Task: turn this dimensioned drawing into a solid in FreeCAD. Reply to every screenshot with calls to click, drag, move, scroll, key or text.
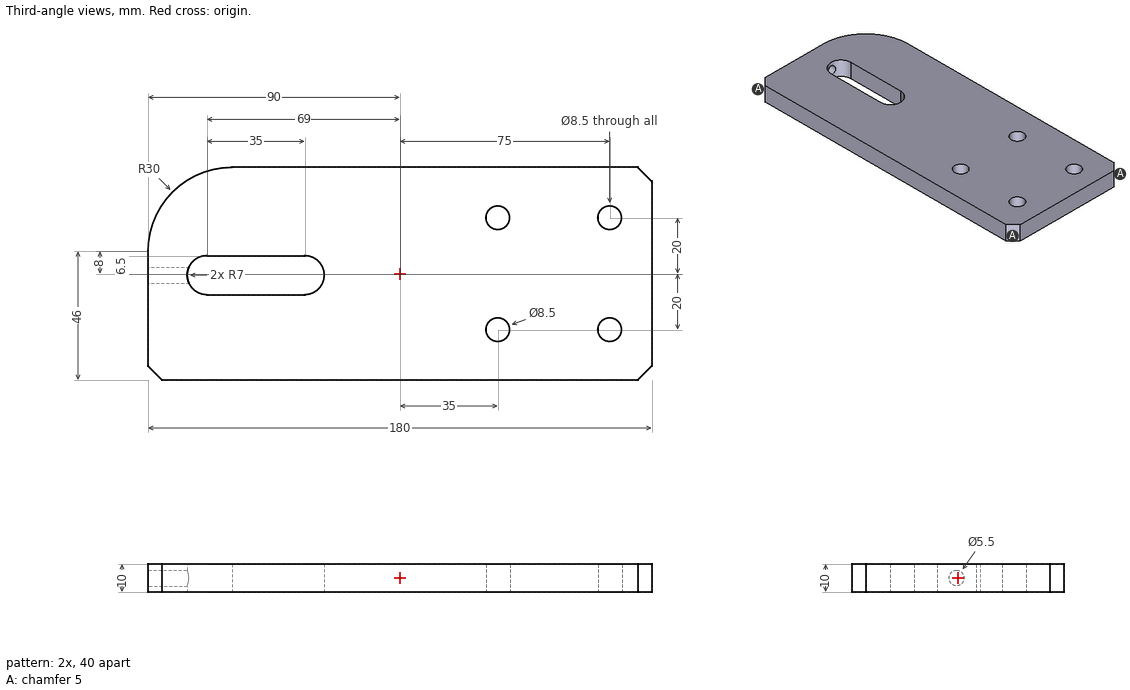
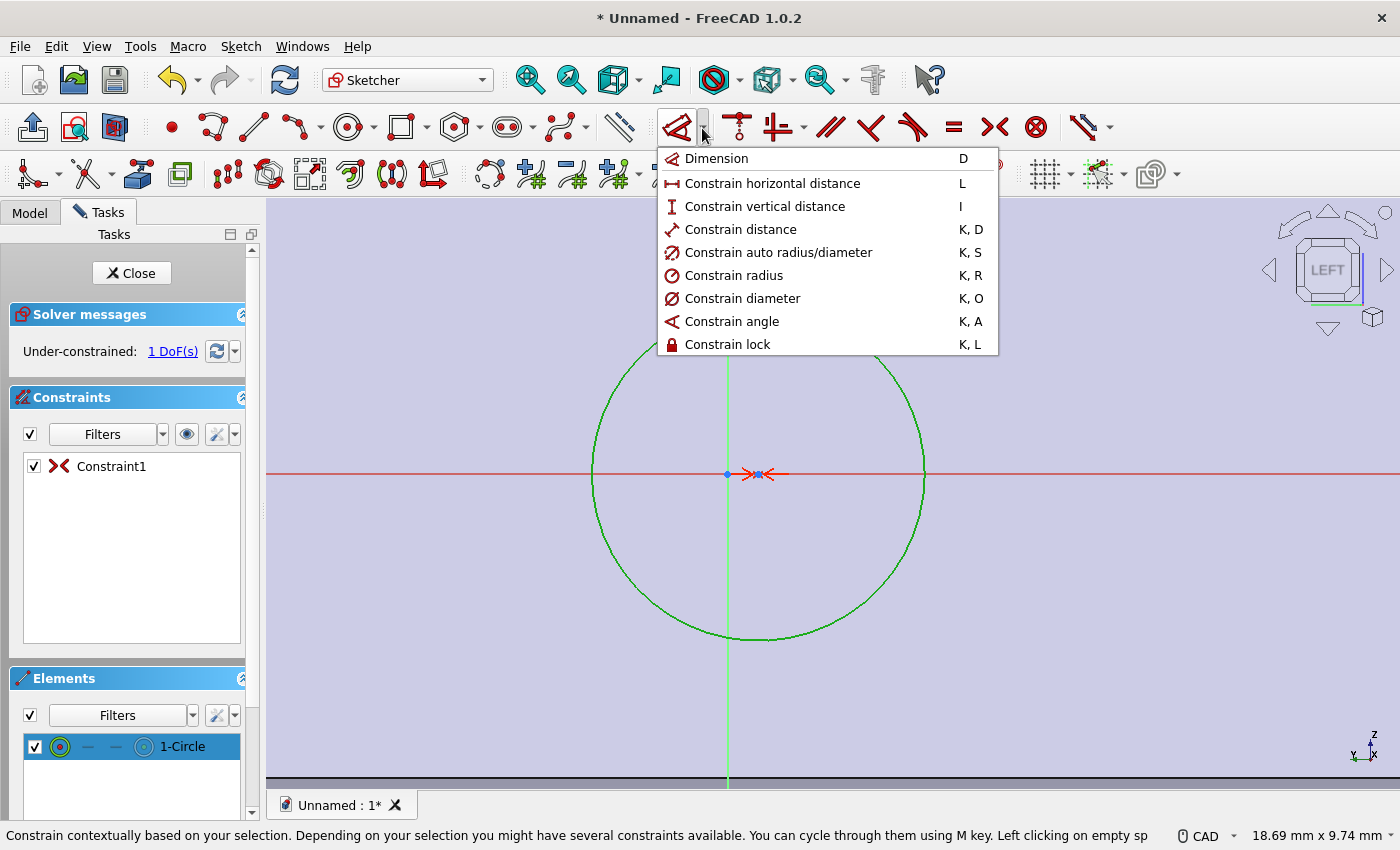
click(828, 298)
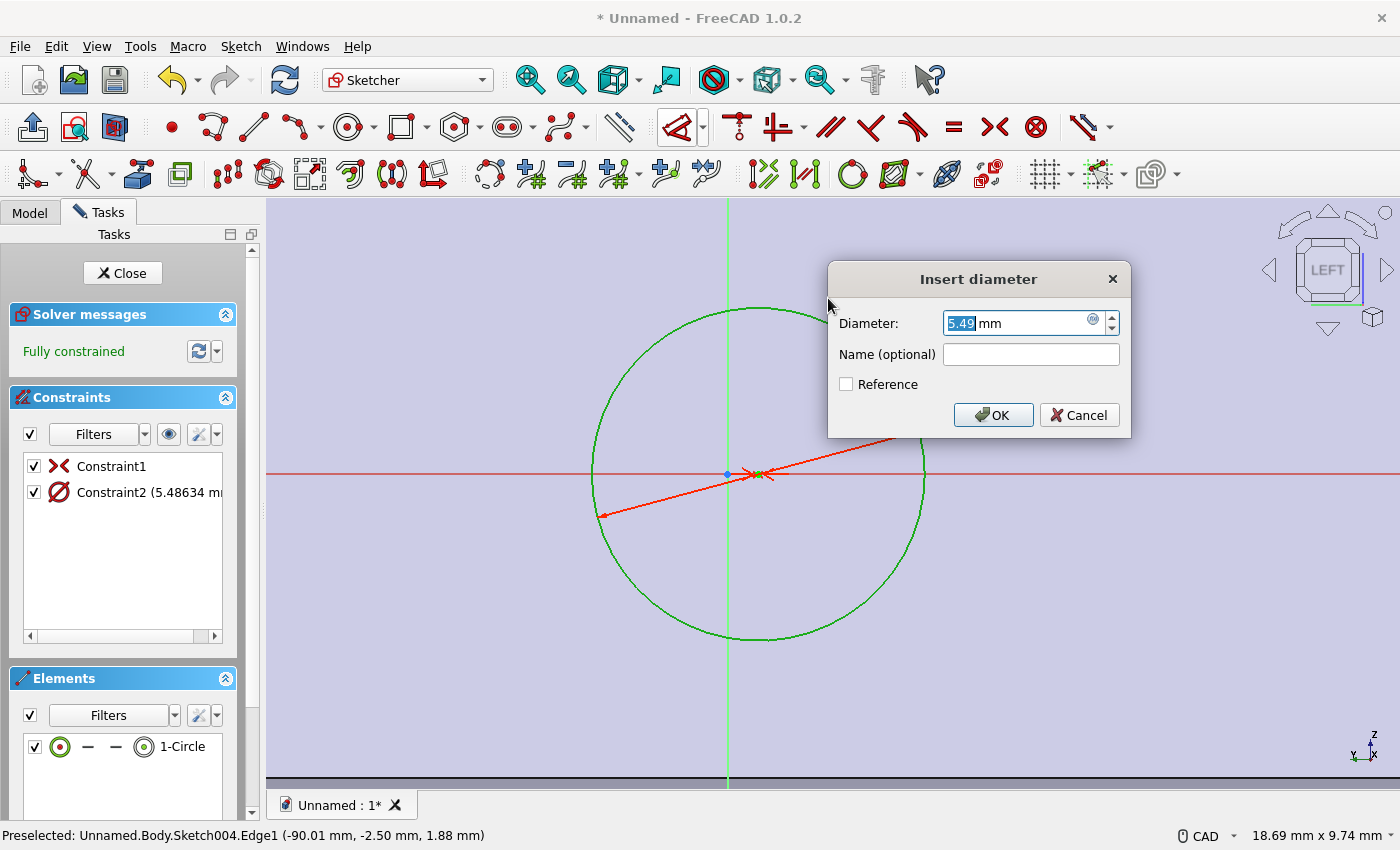
text(5.5)
key(Return)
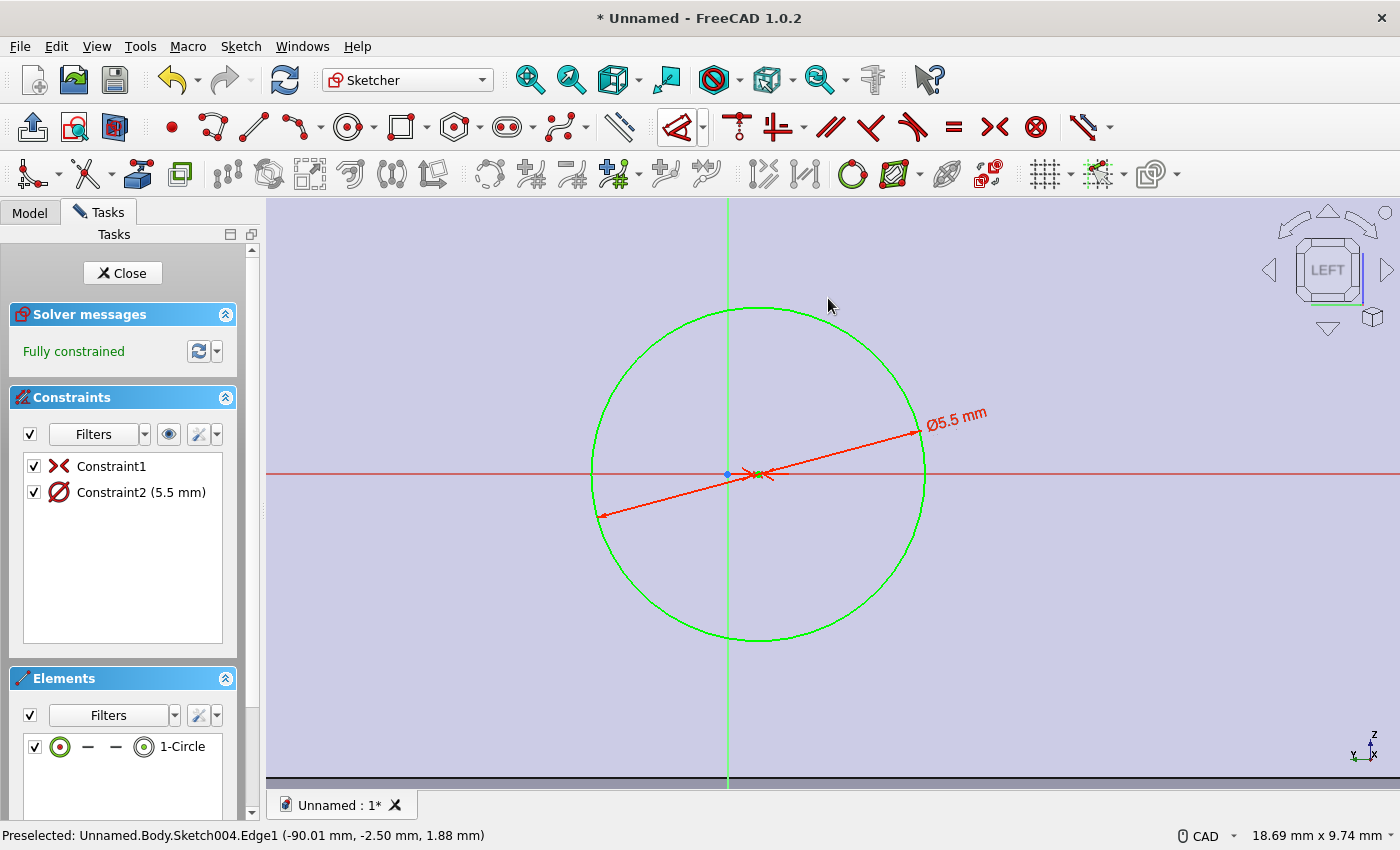
click(123, 273)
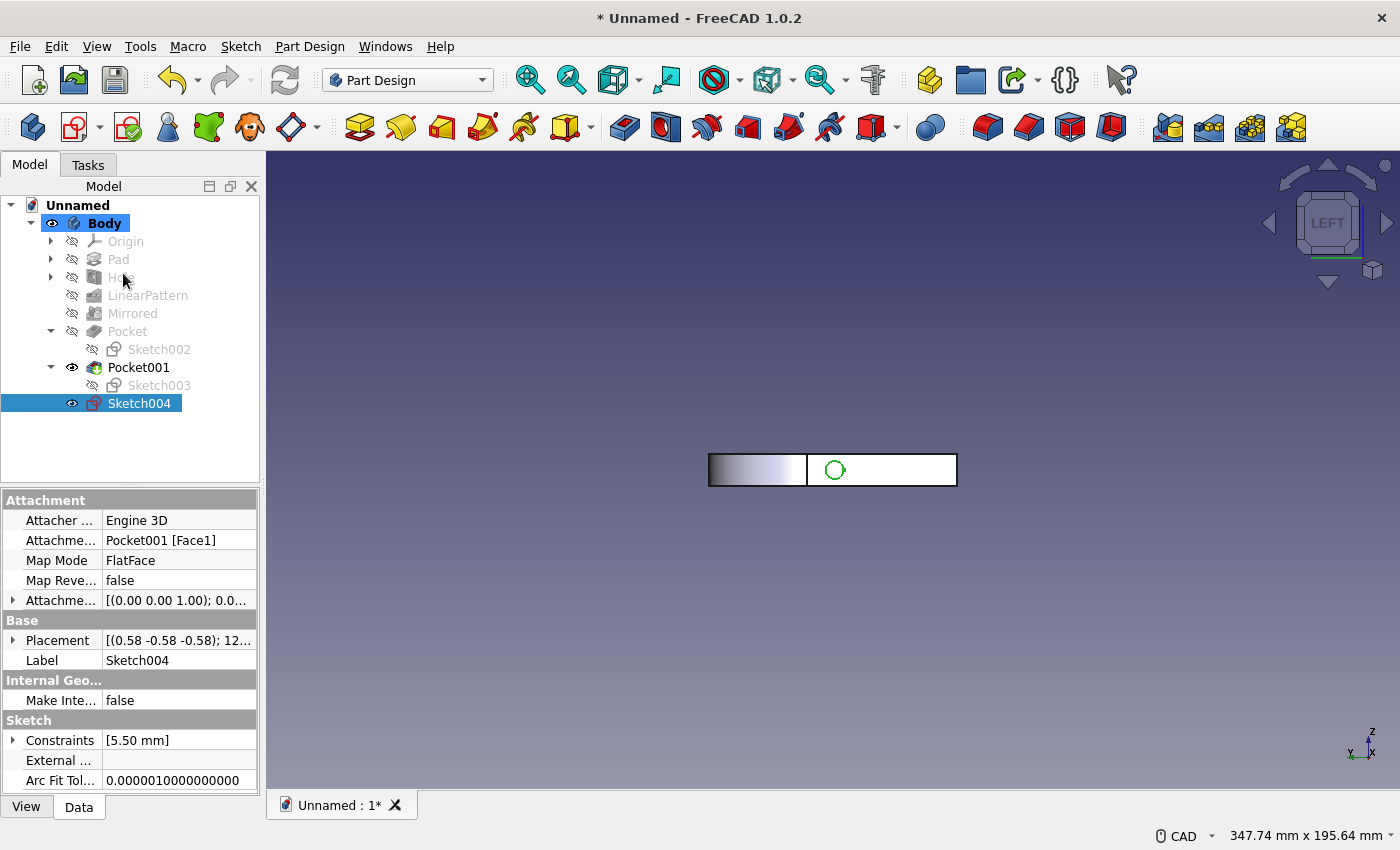
click(625, 128)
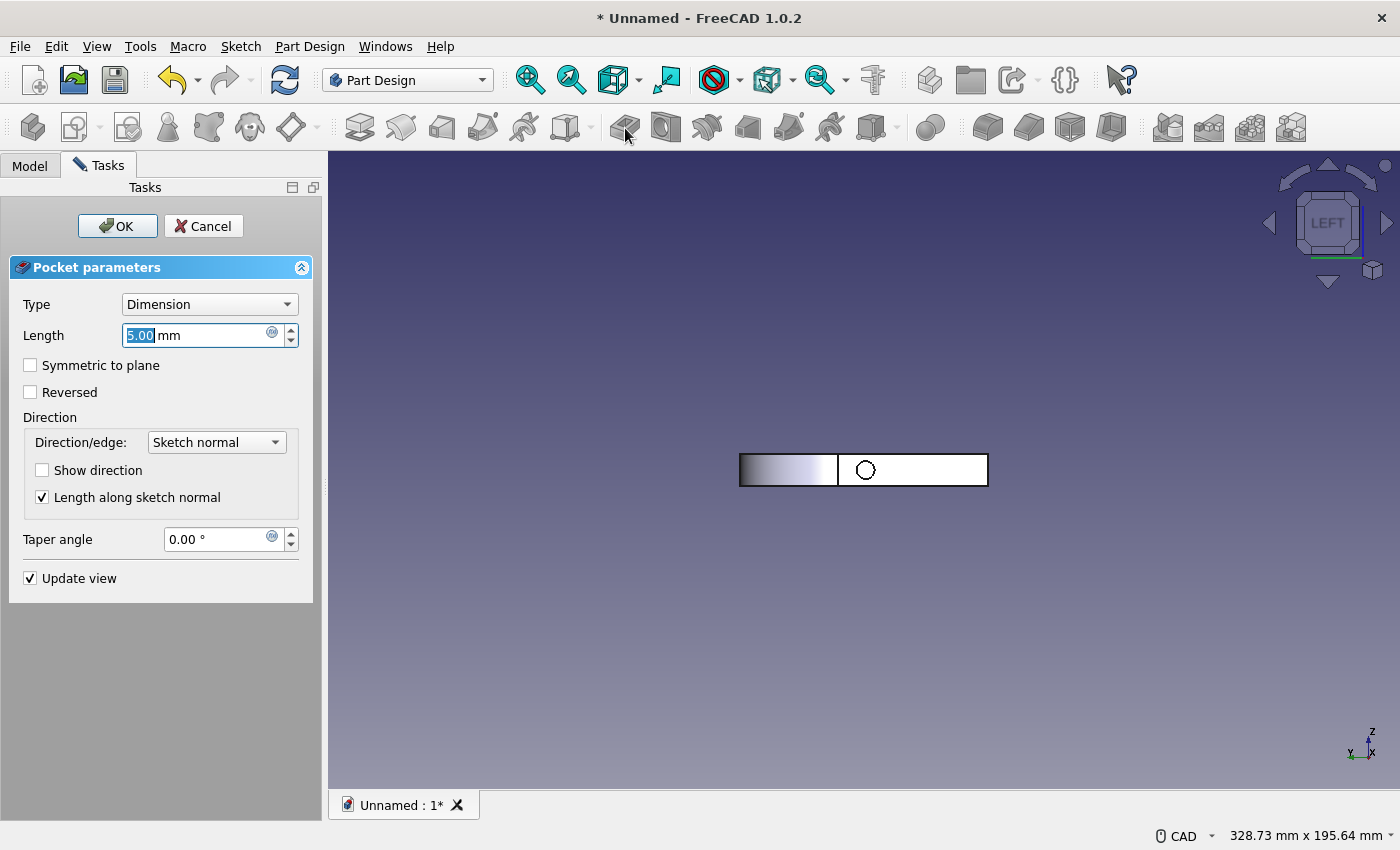
click(210, 304)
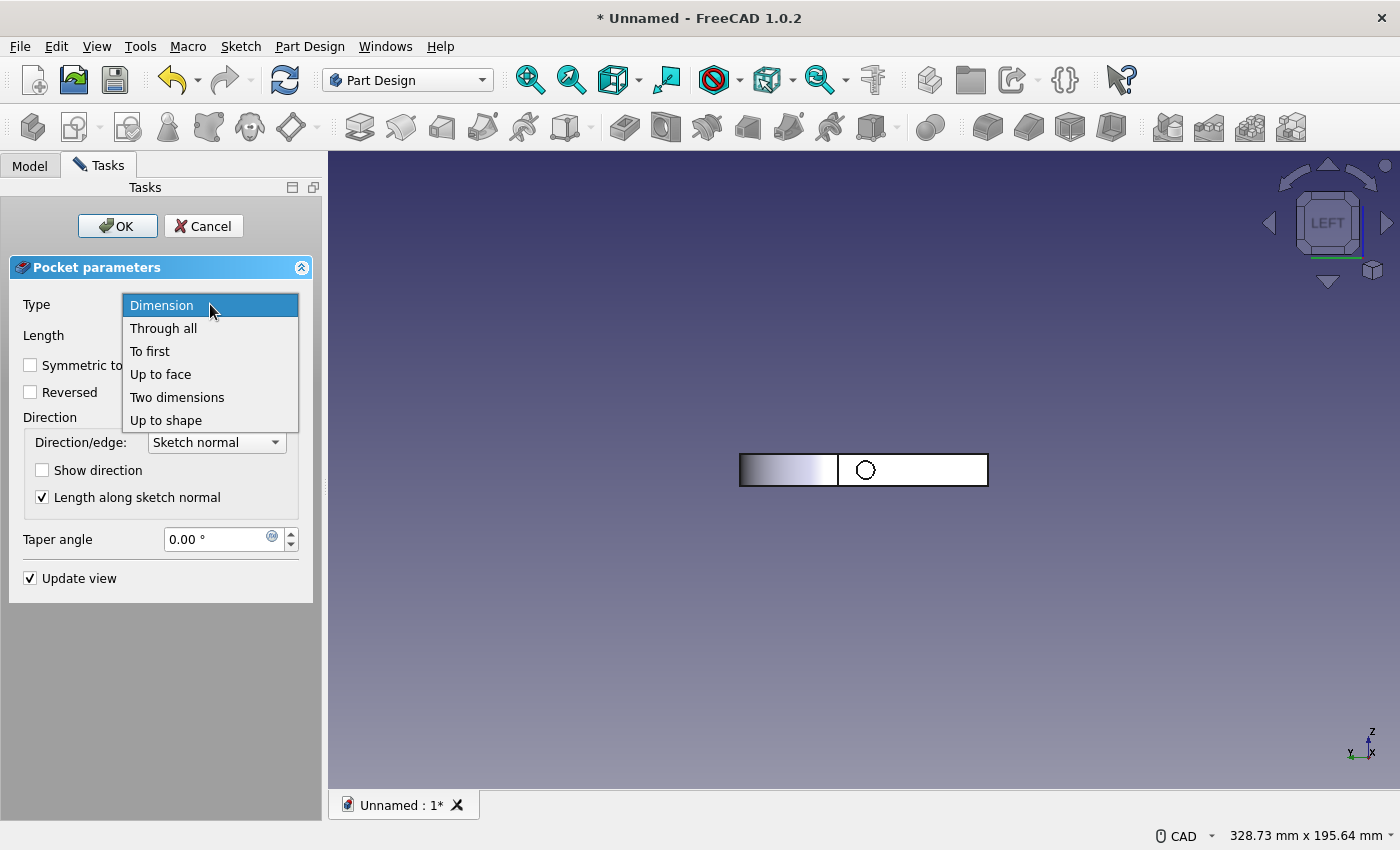
click(208, 352)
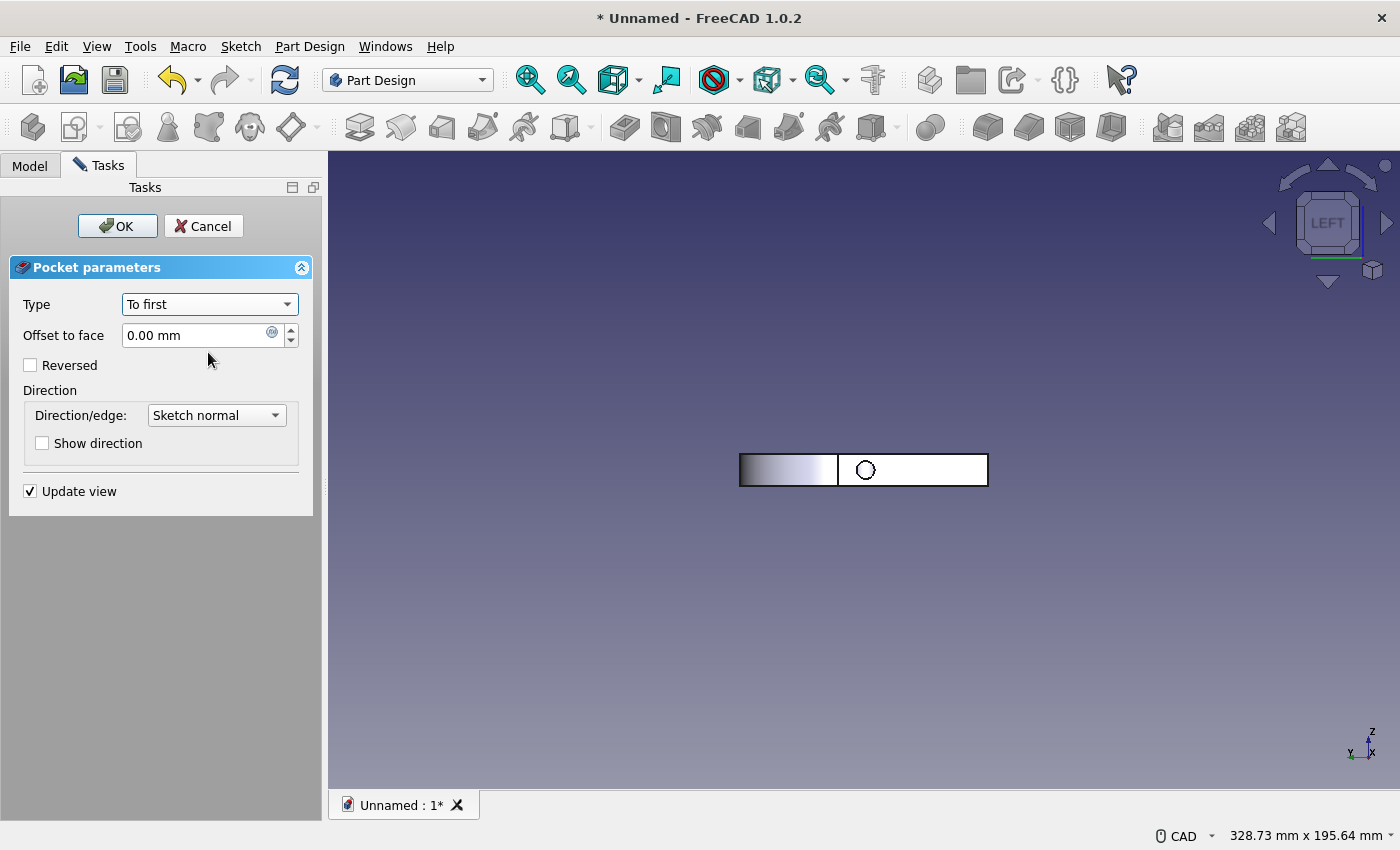
click(118, 226)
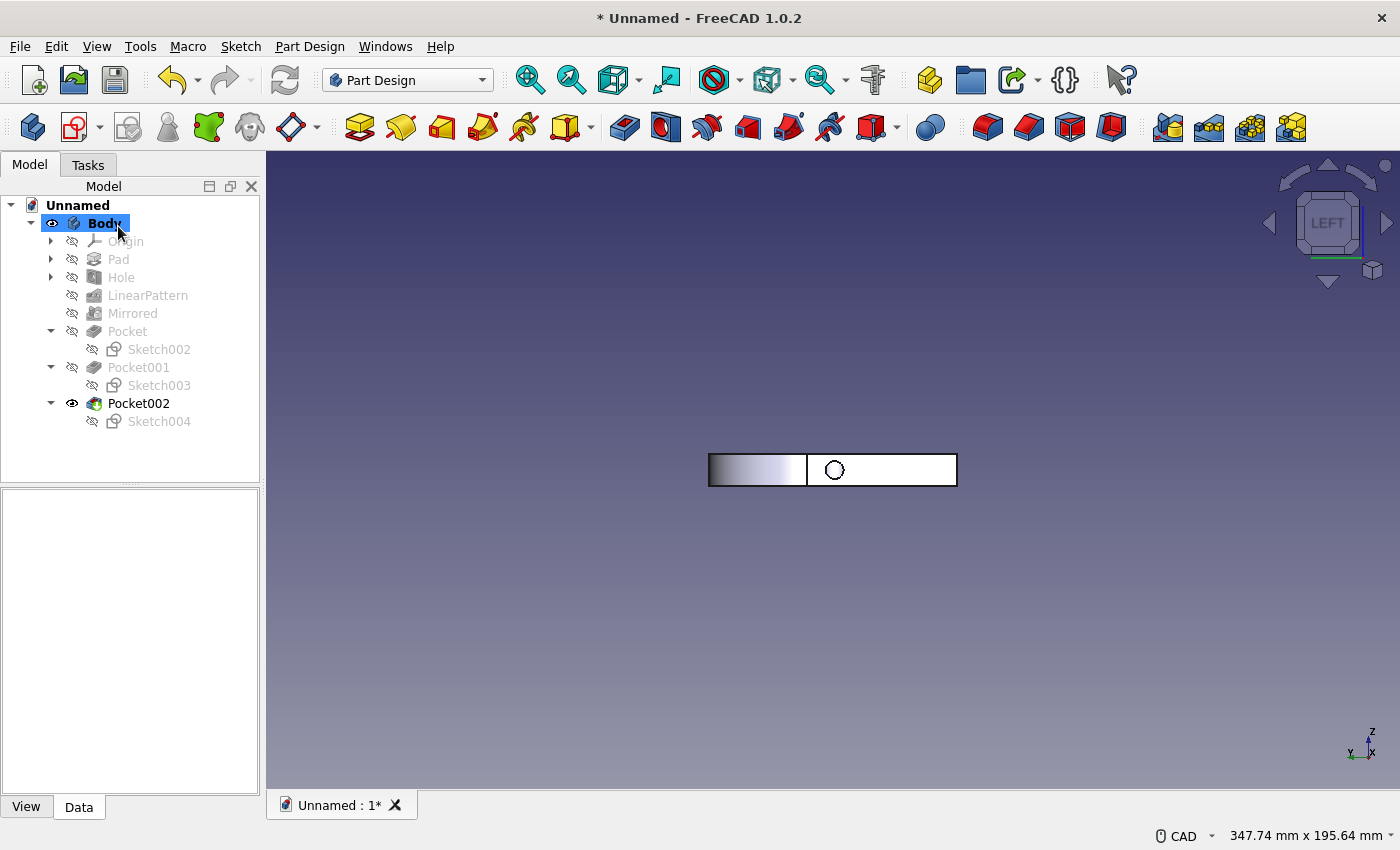
click(531, 80)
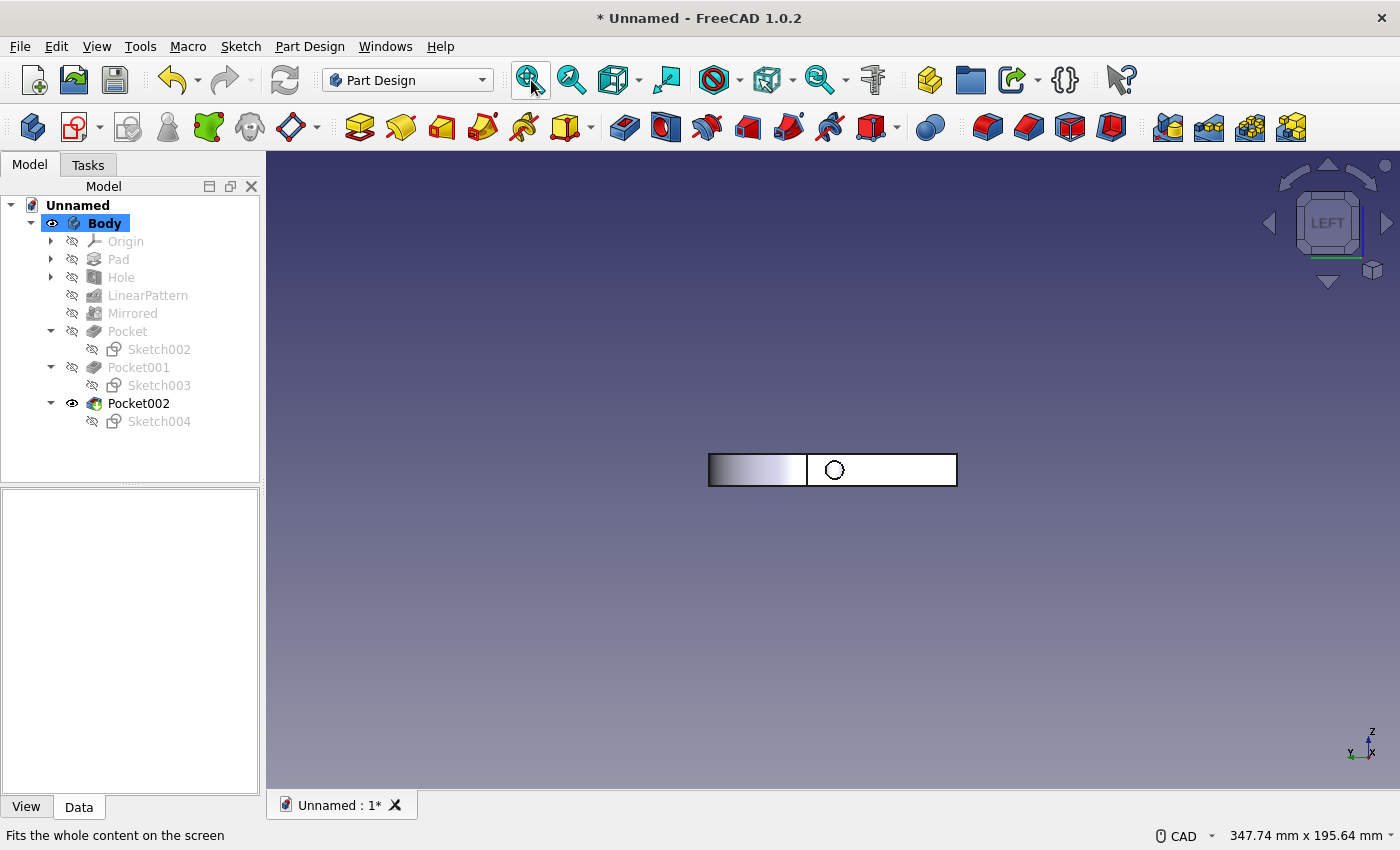
click(957, 469)